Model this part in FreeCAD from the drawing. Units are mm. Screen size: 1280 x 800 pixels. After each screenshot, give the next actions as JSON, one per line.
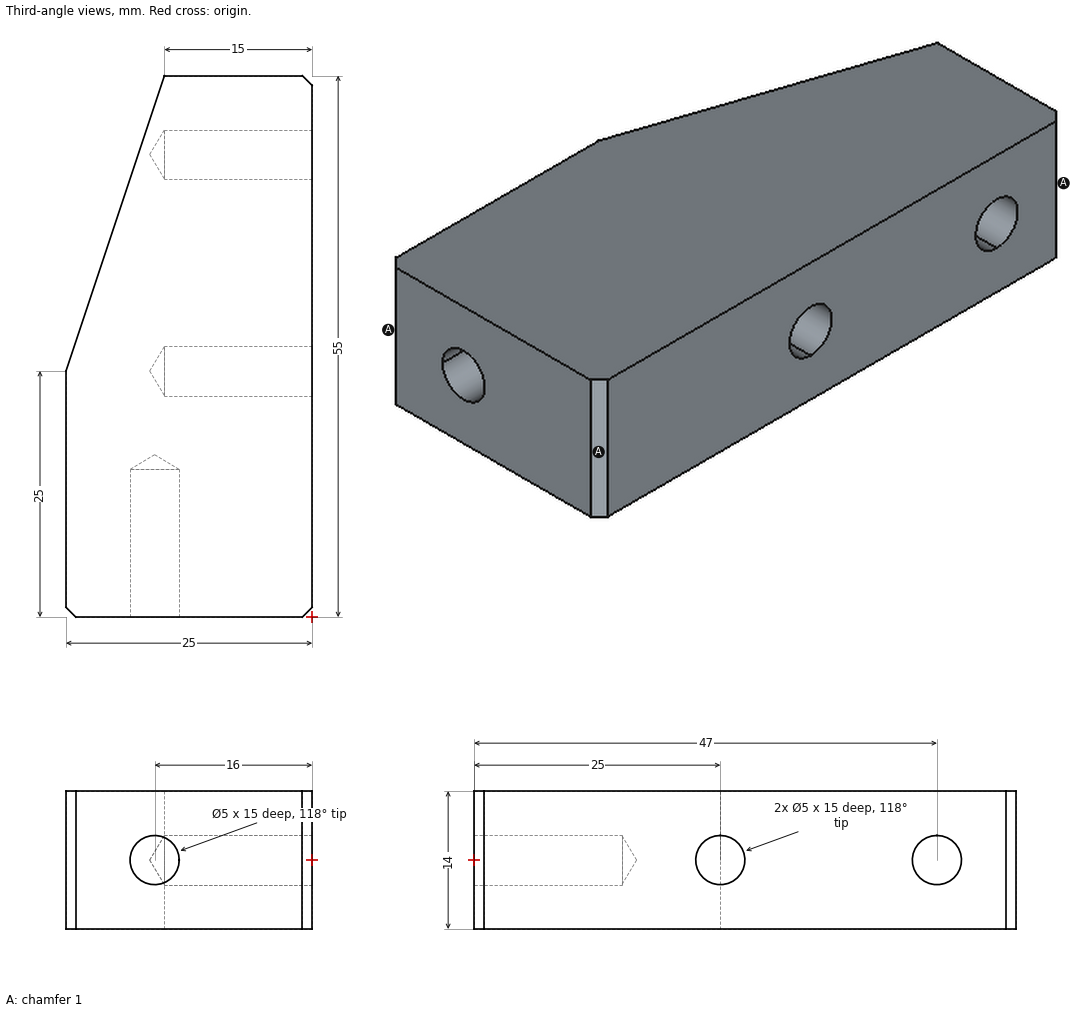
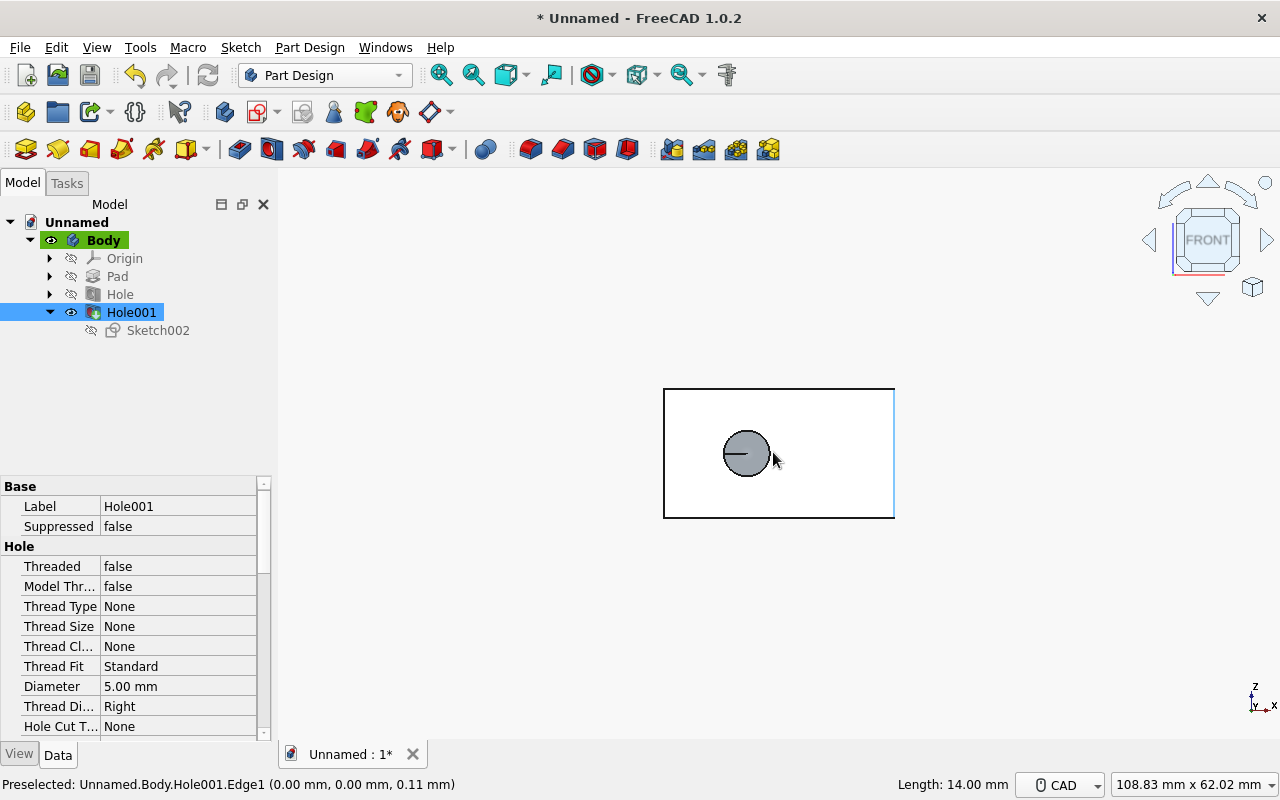
{"action": "left_click", "coordinate": [664, 453], "text": "ctrl"}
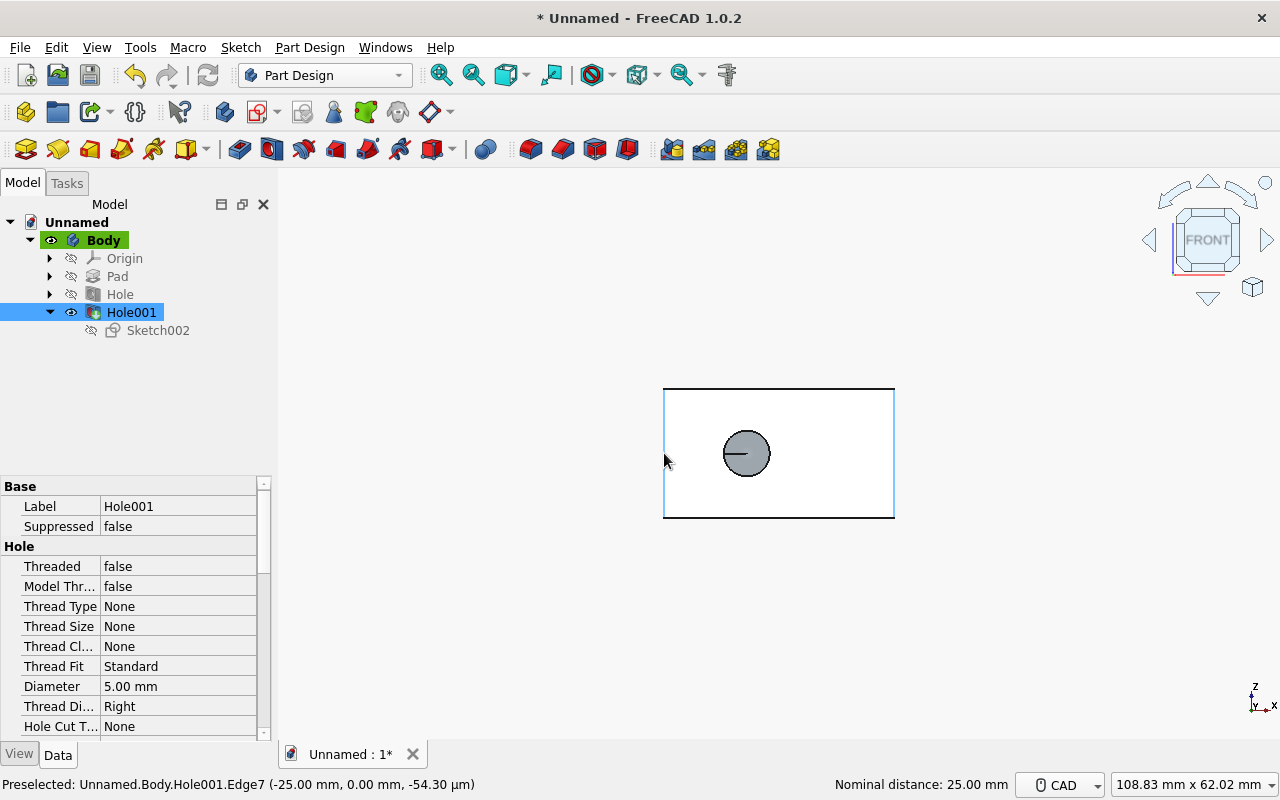
{"action": "key", "text": "3"}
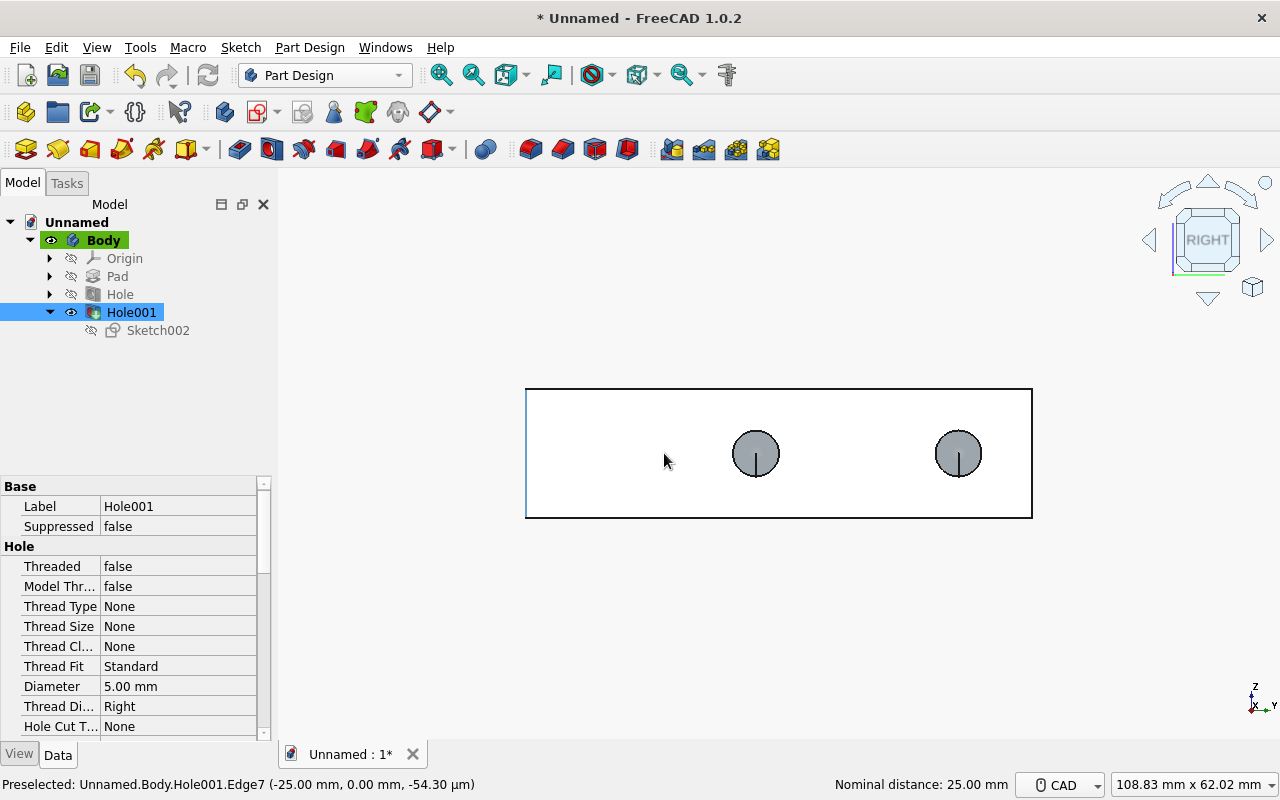
{"action": "left_click", "coordinate": [1032, 452], "text": "ctrl"}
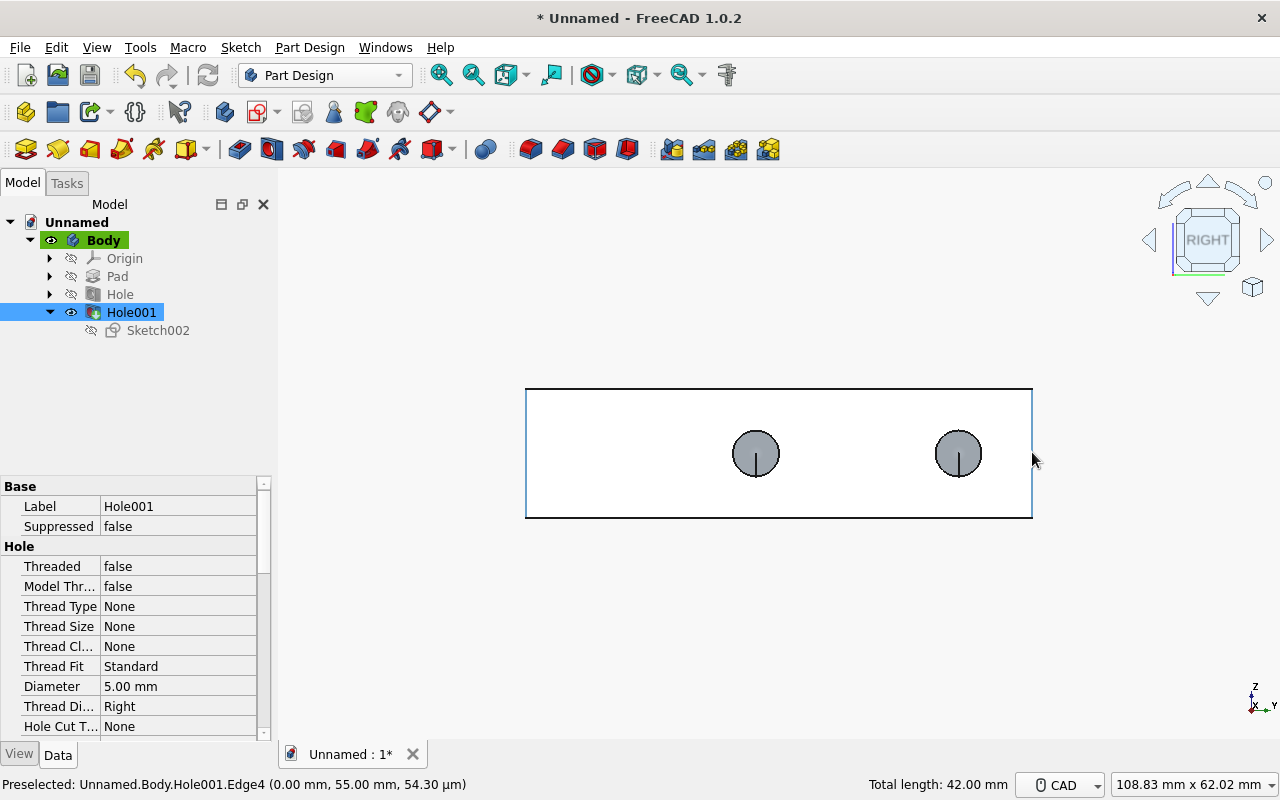
{"action": "left_click", "coordinate": [564, 150]}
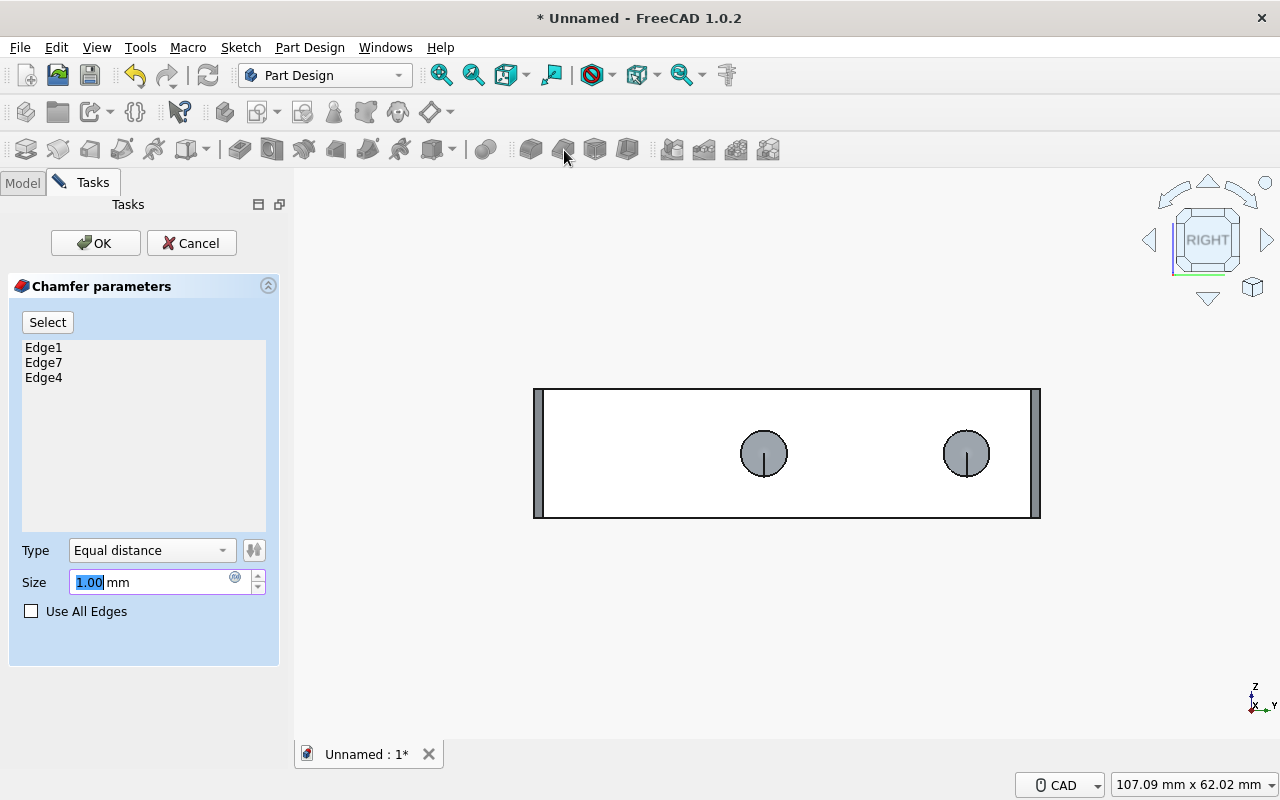
{"action": "type", "text": "1"}
{"action": "key", "text": "Tab"}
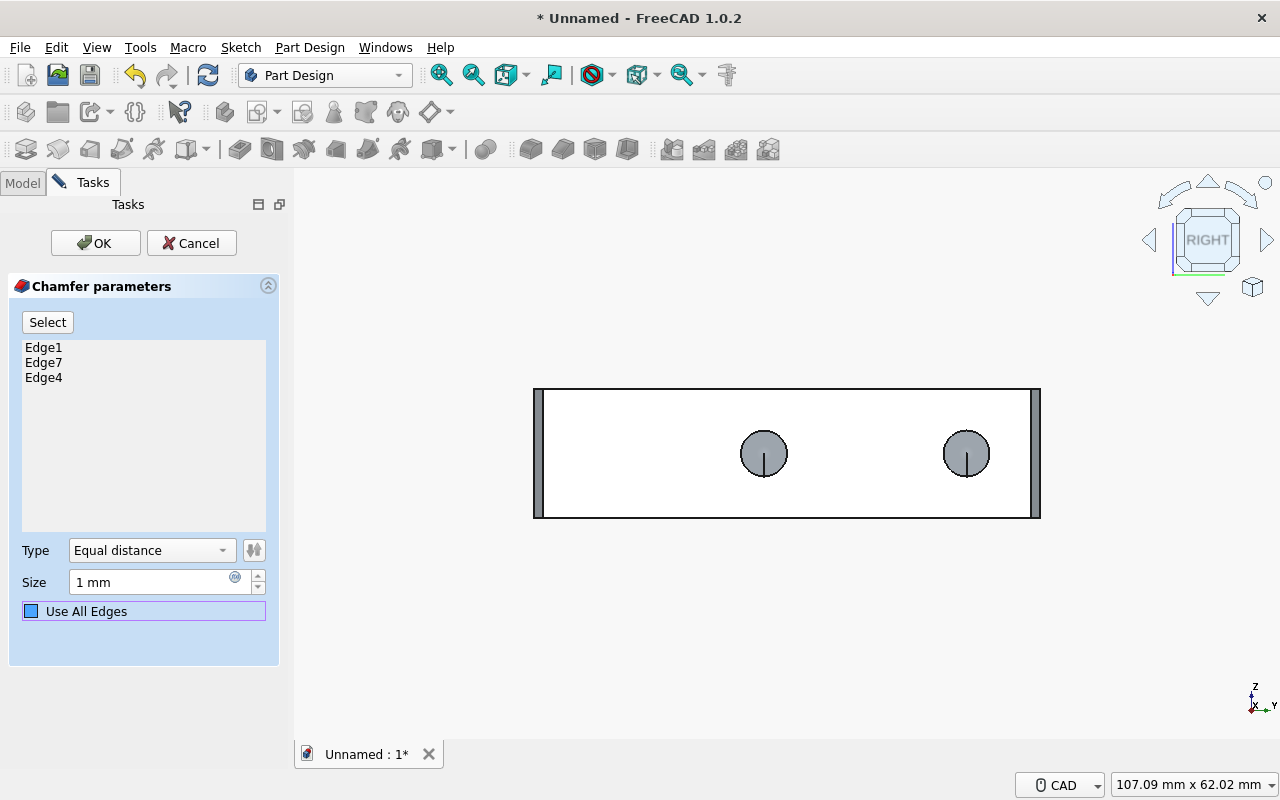
{"action": "left_click", "coordinate": [96, 243]}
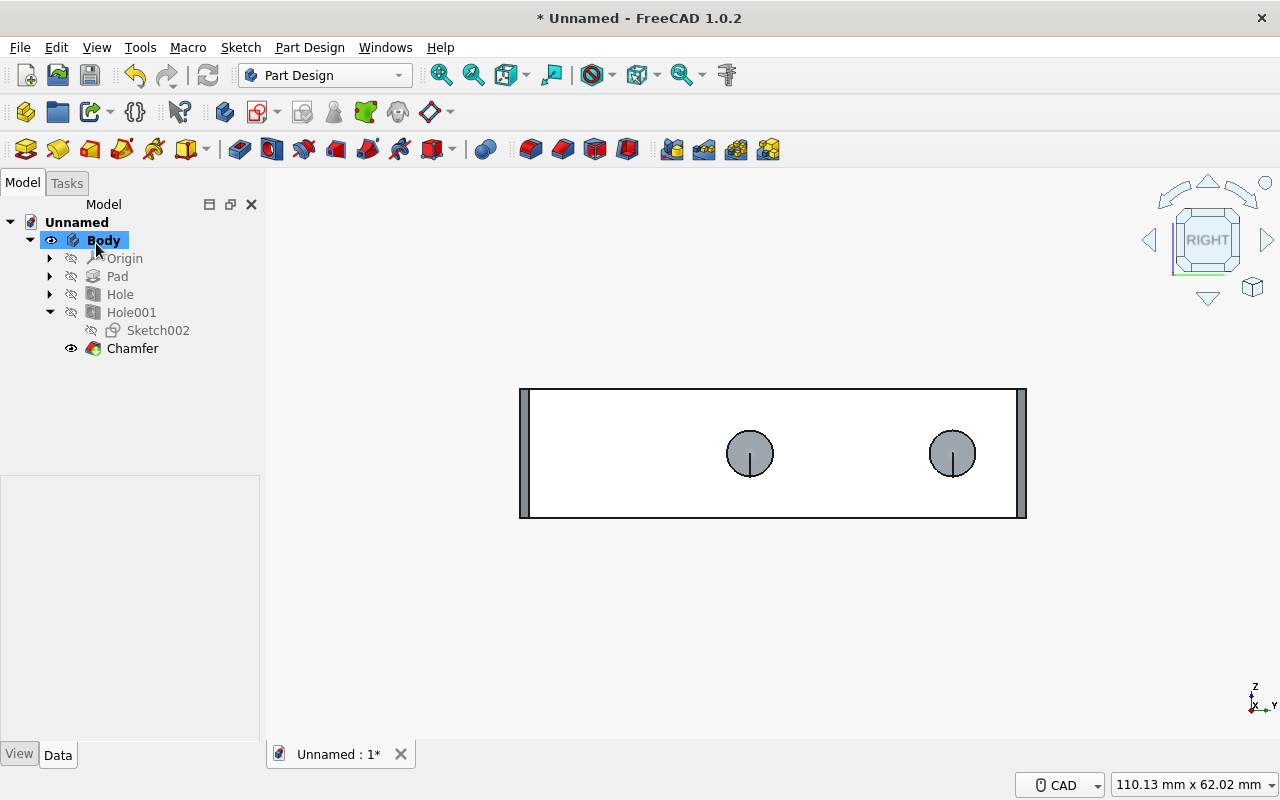
{"action": "key", "text": "0"}